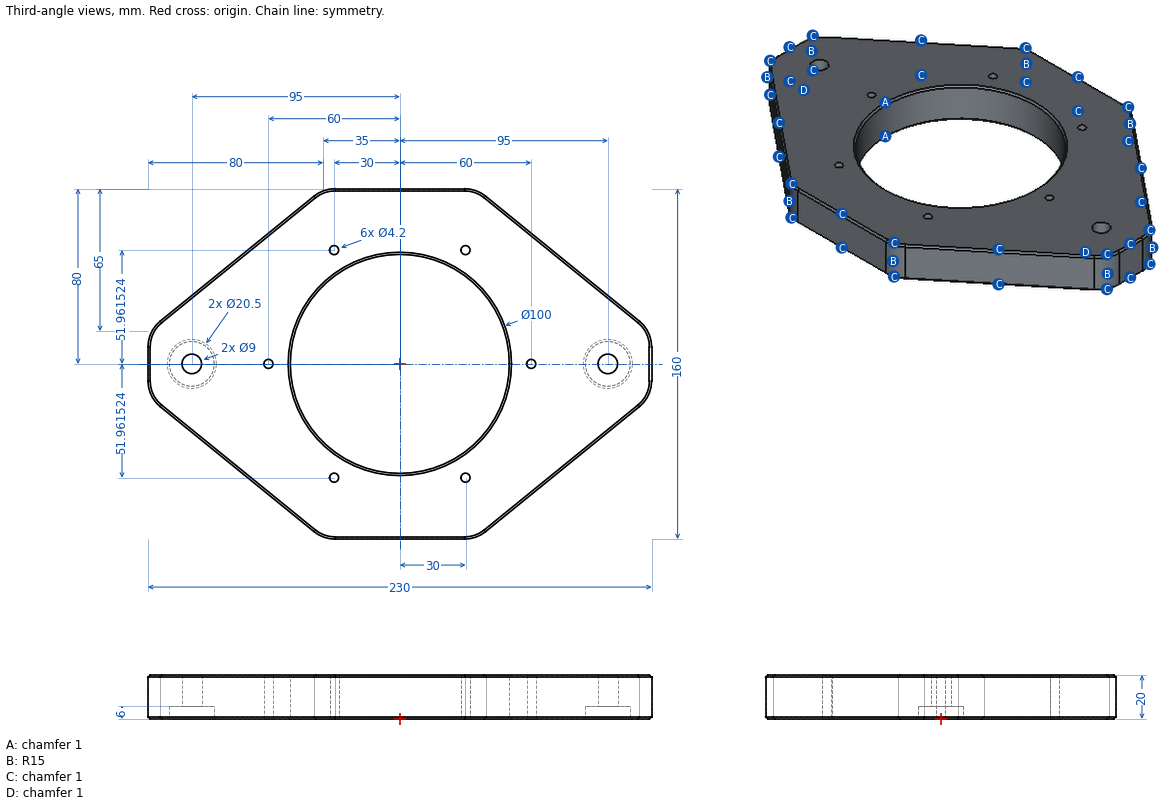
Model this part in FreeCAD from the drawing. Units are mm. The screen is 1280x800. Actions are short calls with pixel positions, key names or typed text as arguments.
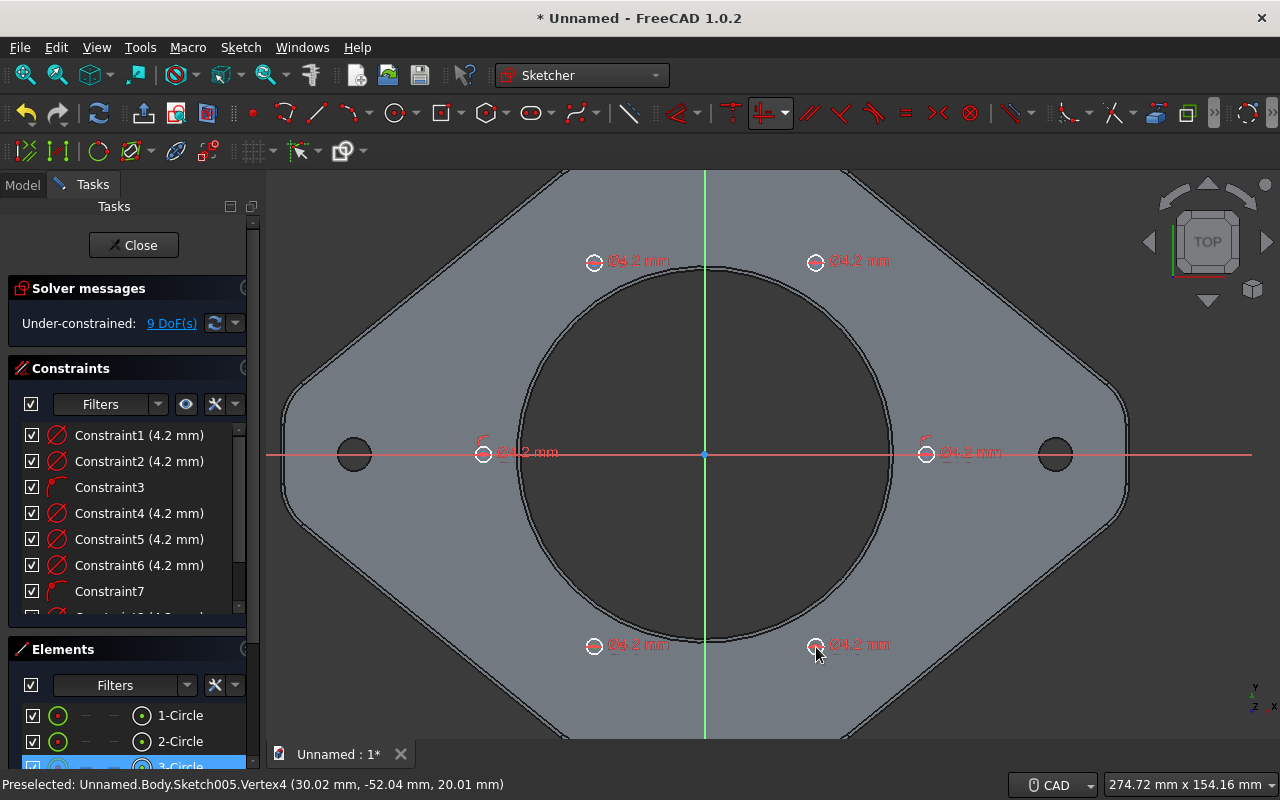
click(788, 114)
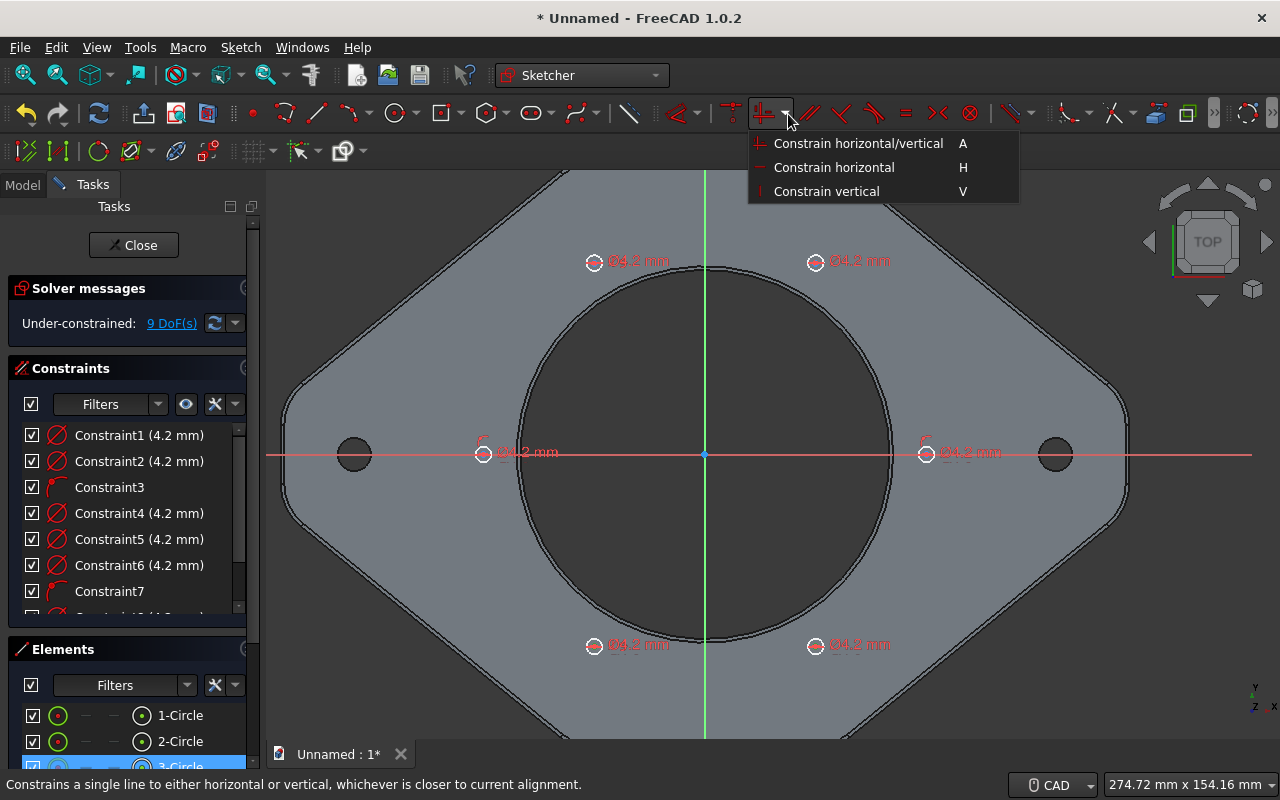
click(884, 167)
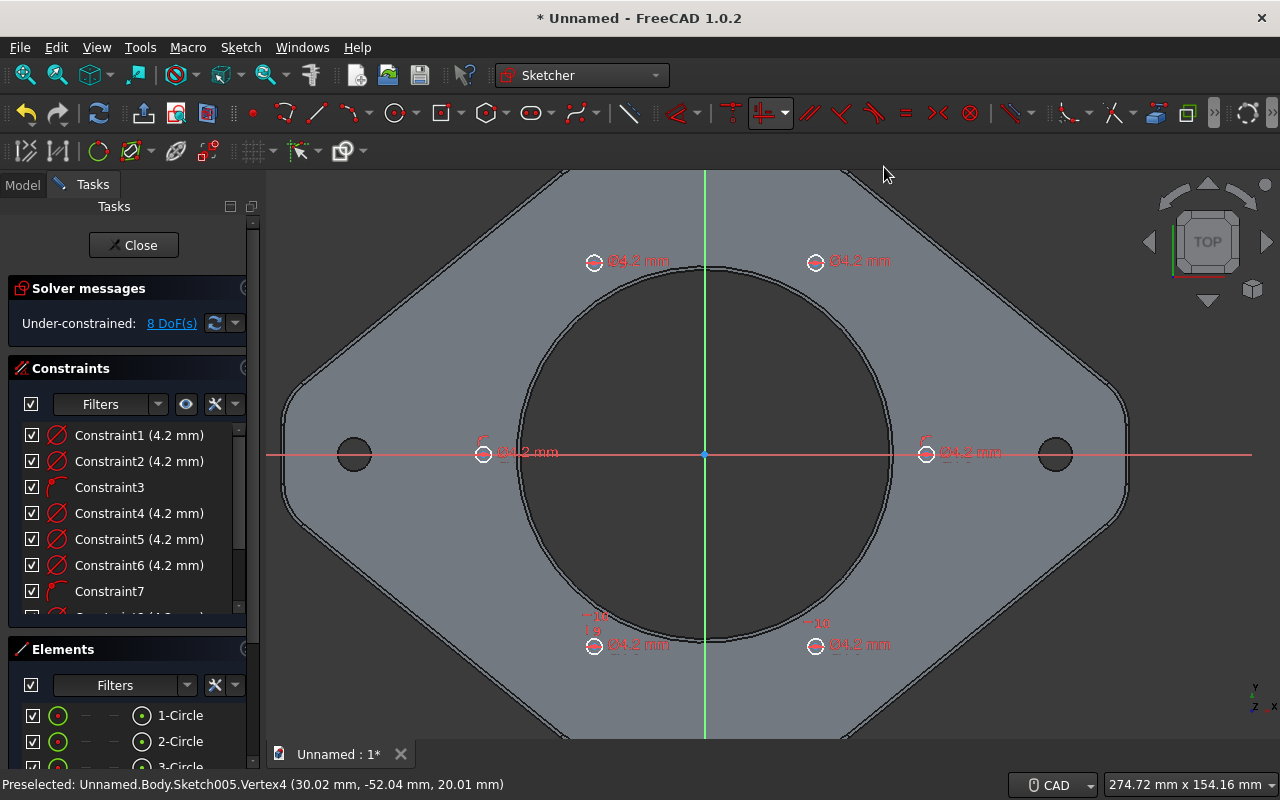
click(816, 647)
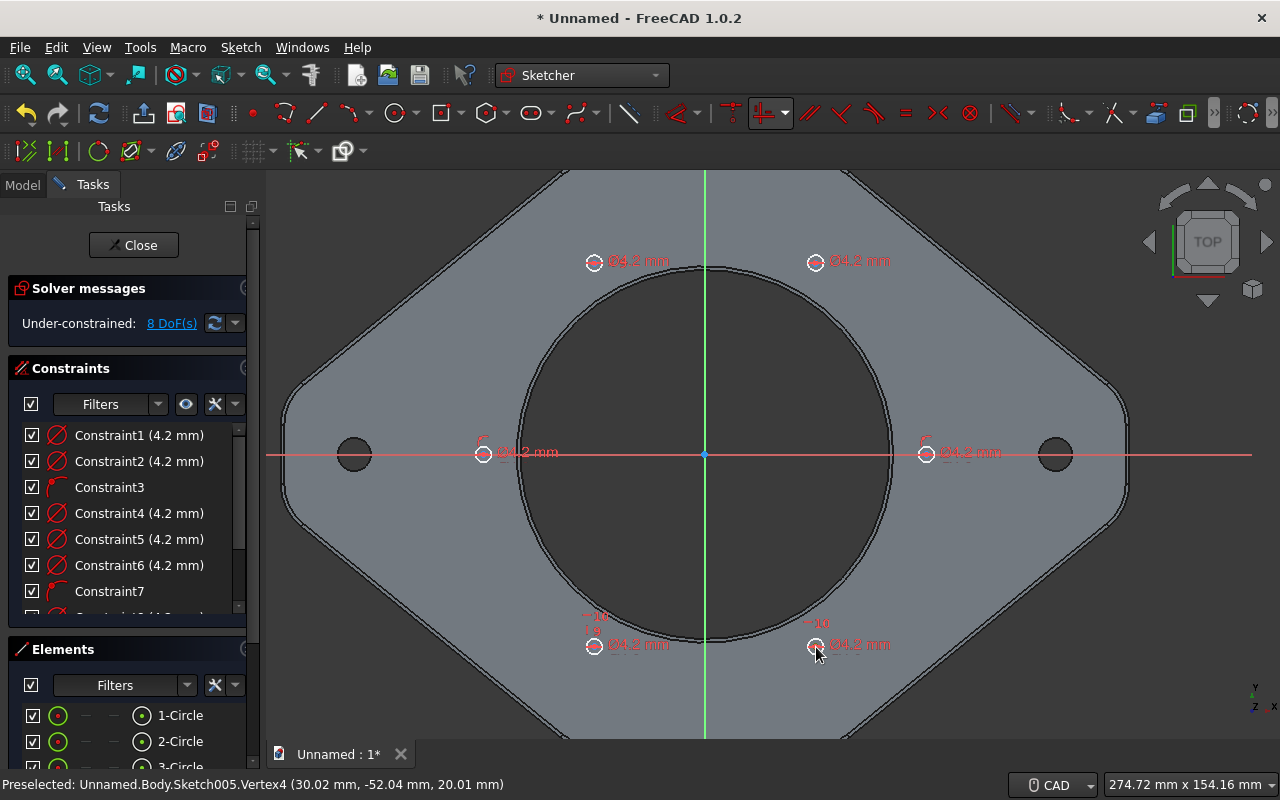
click(816, 263)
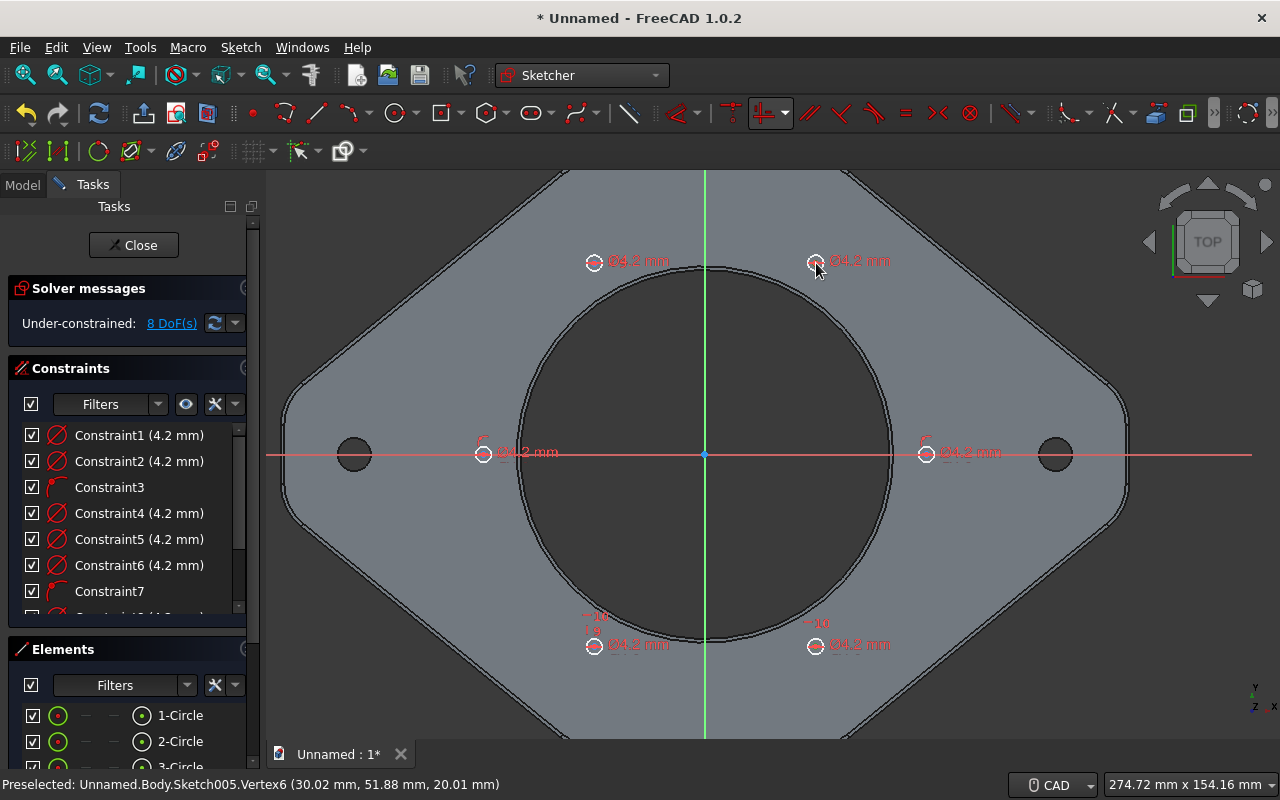
click(788, 114)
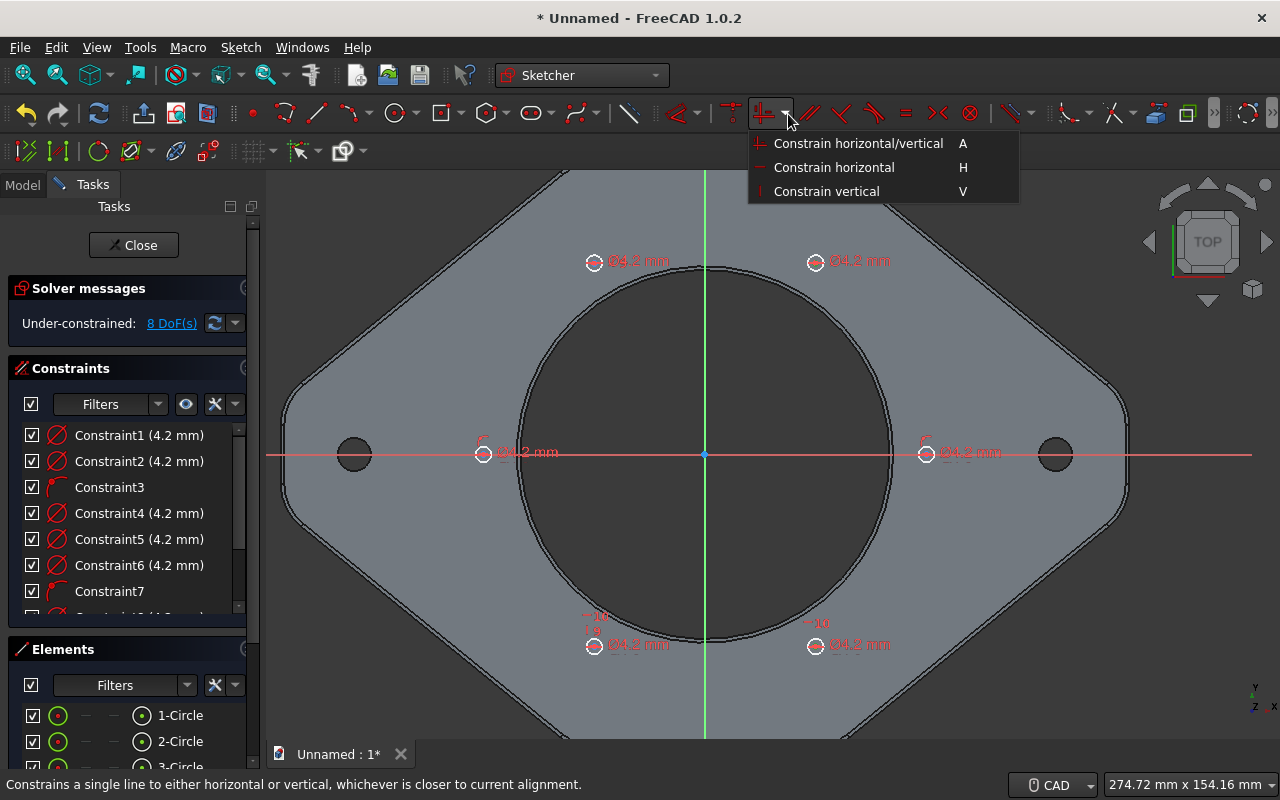
click(884, 191)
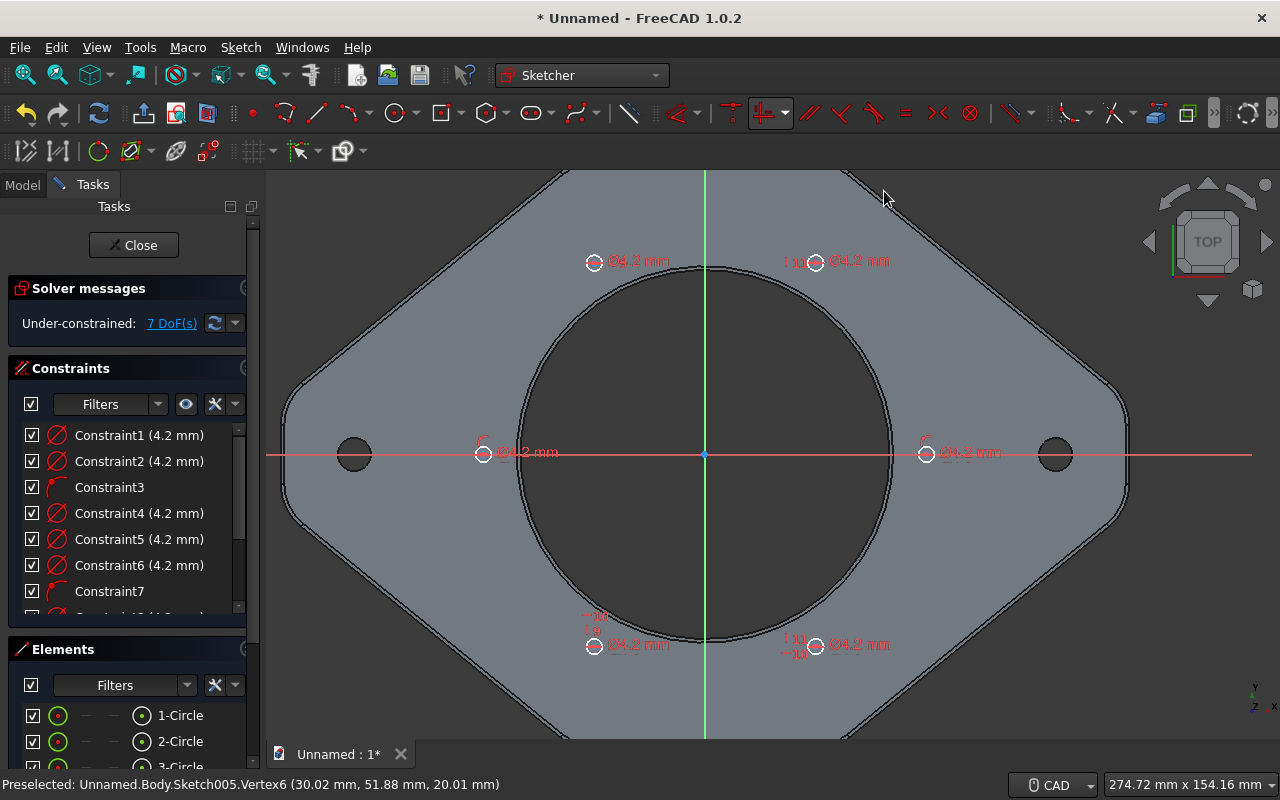
click(594, 263)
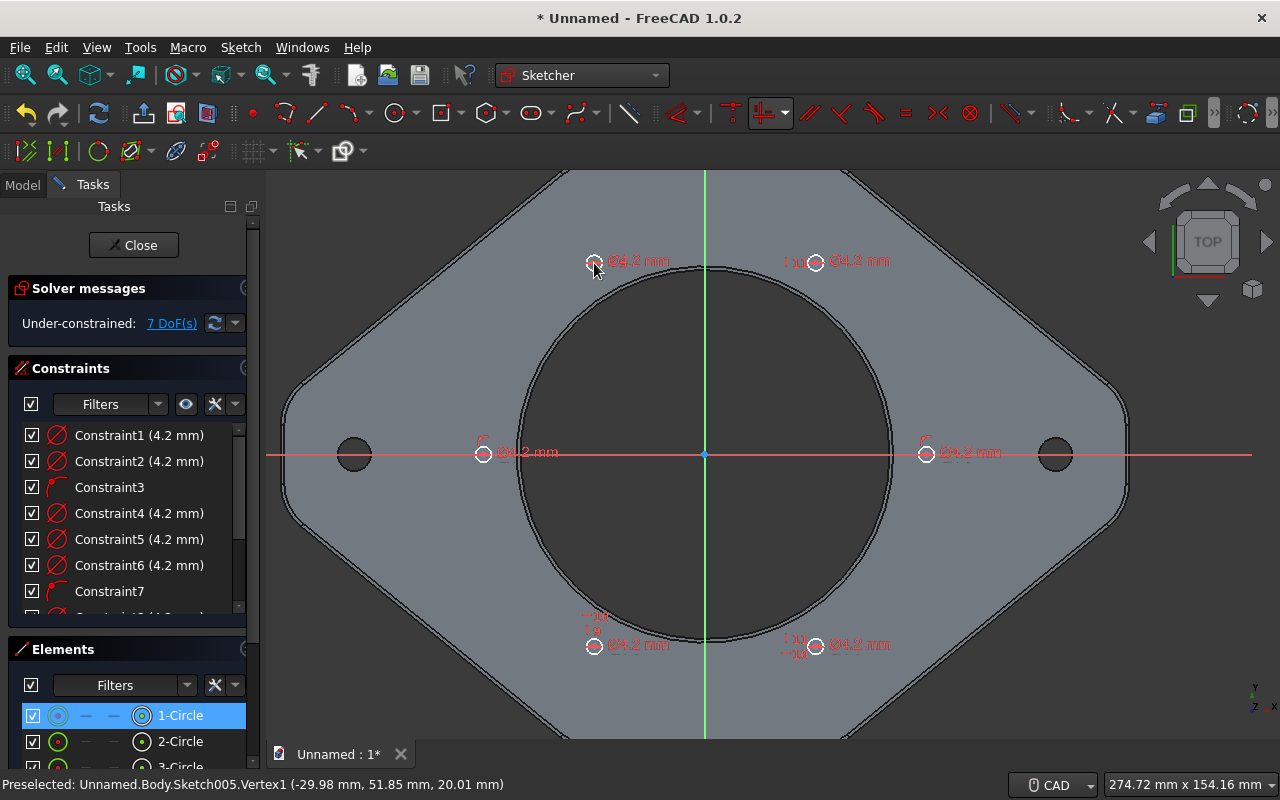
click(816, 263)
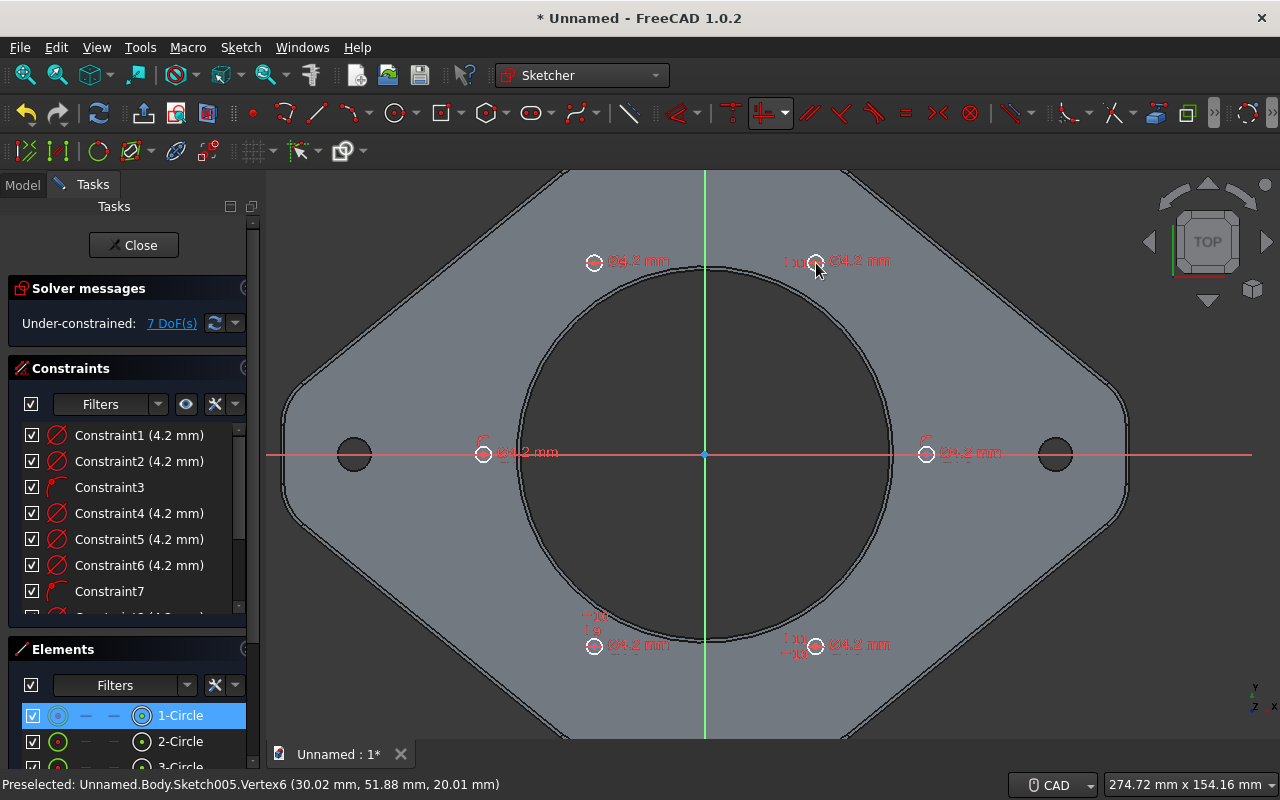
click(788, 114)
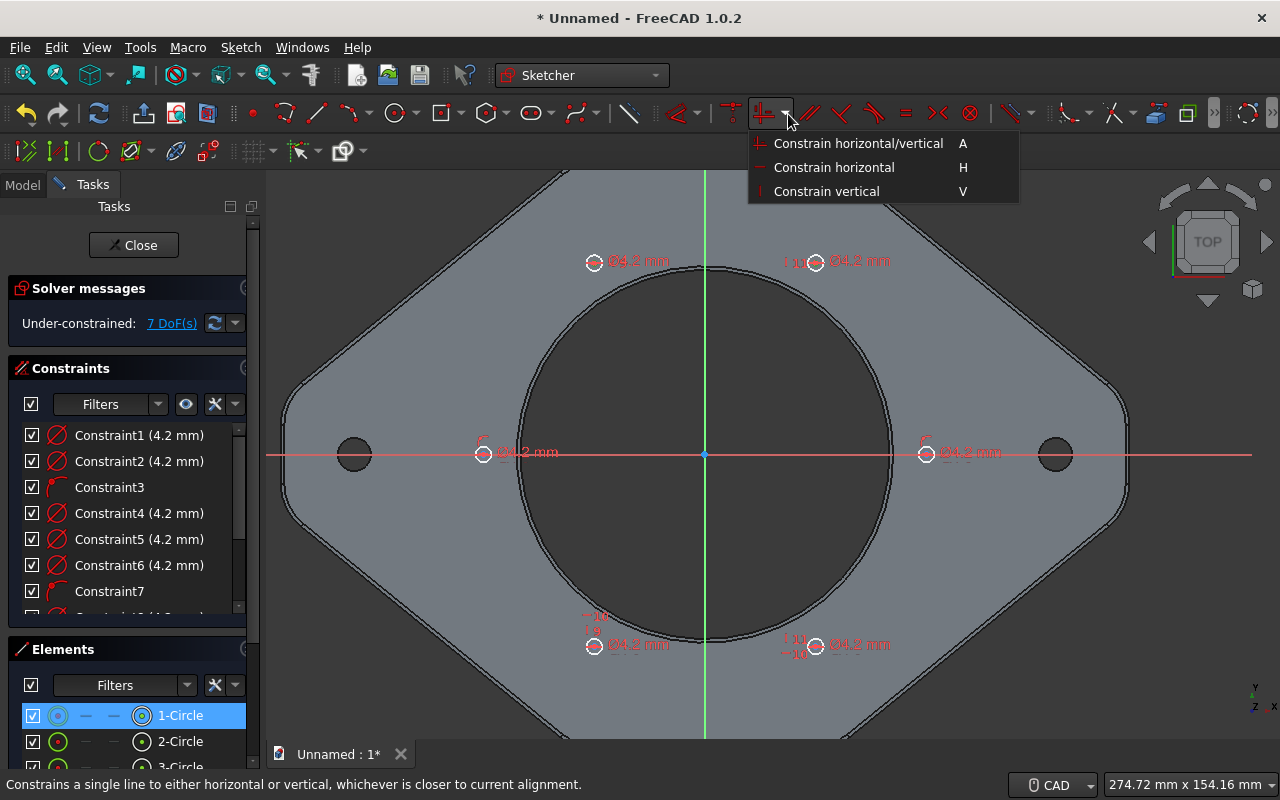
click(884, 167)